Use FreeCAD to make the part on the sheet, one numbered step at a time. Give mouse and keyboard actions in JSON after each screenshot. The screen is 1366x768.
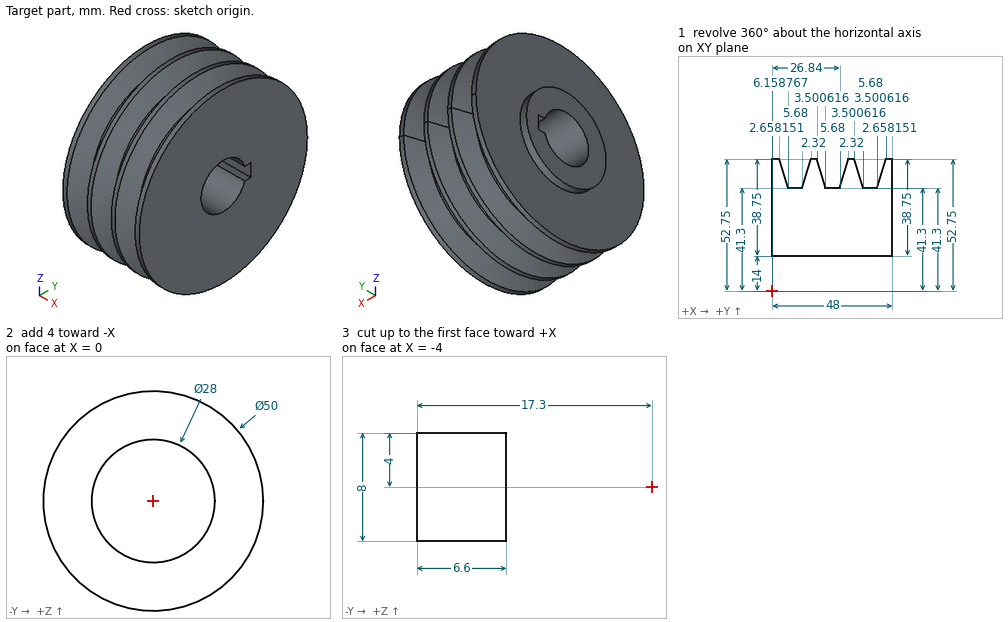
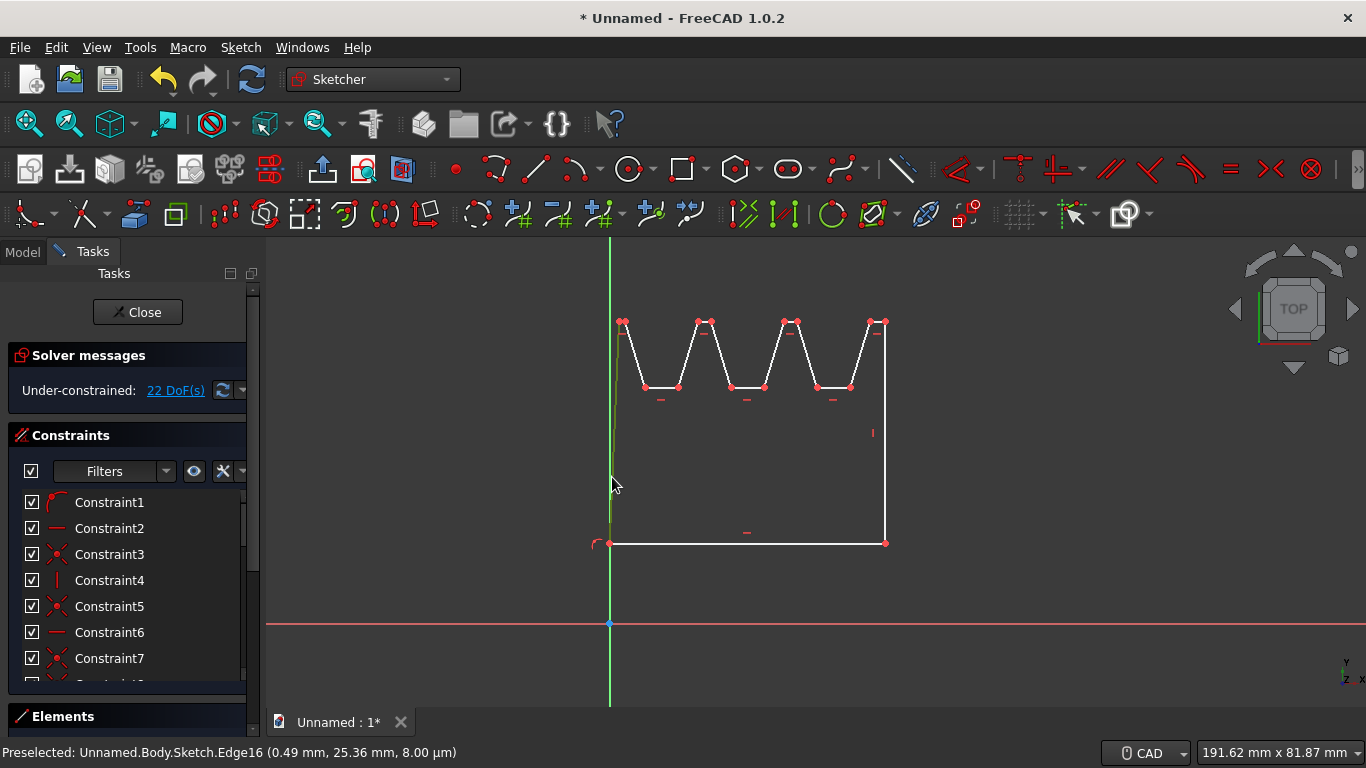
{"action": "key", "text": "v"}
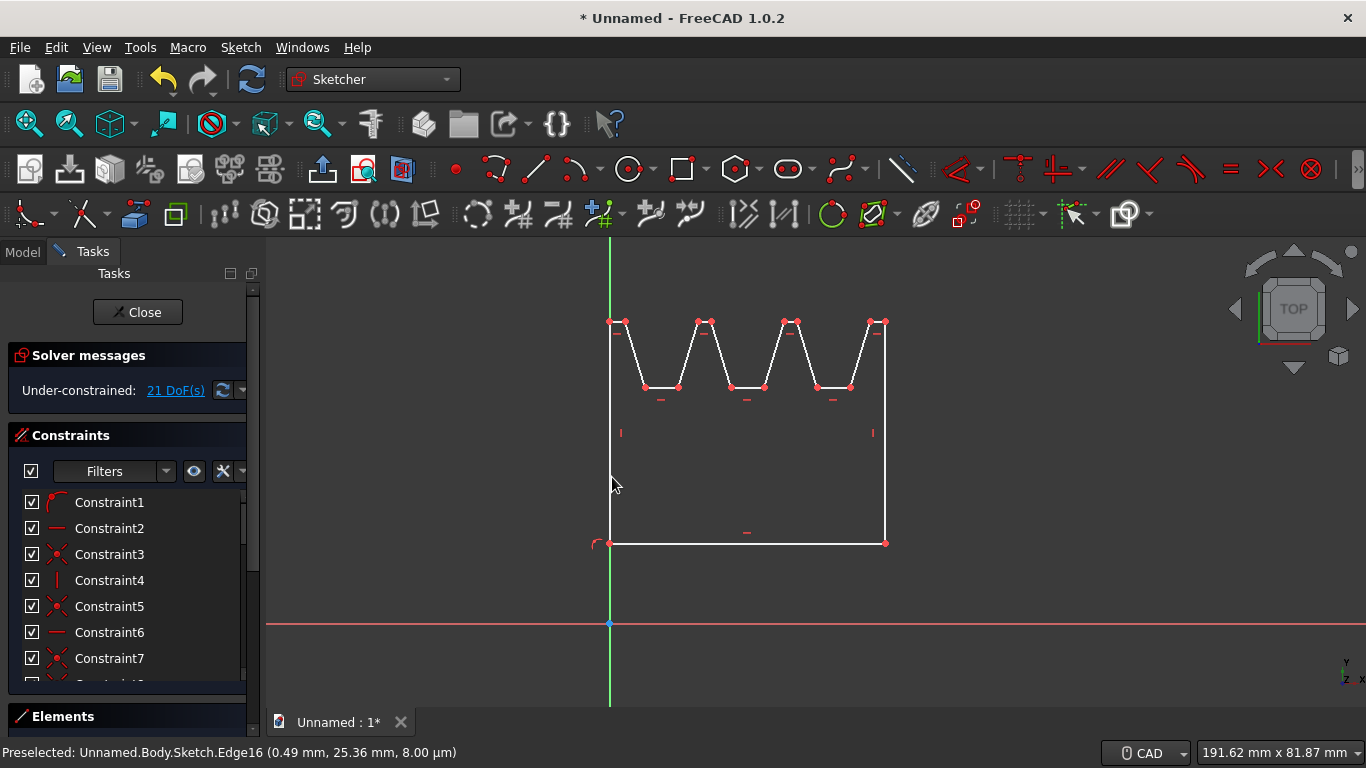
{"action": "left_click", "coordinate": [956, 170]}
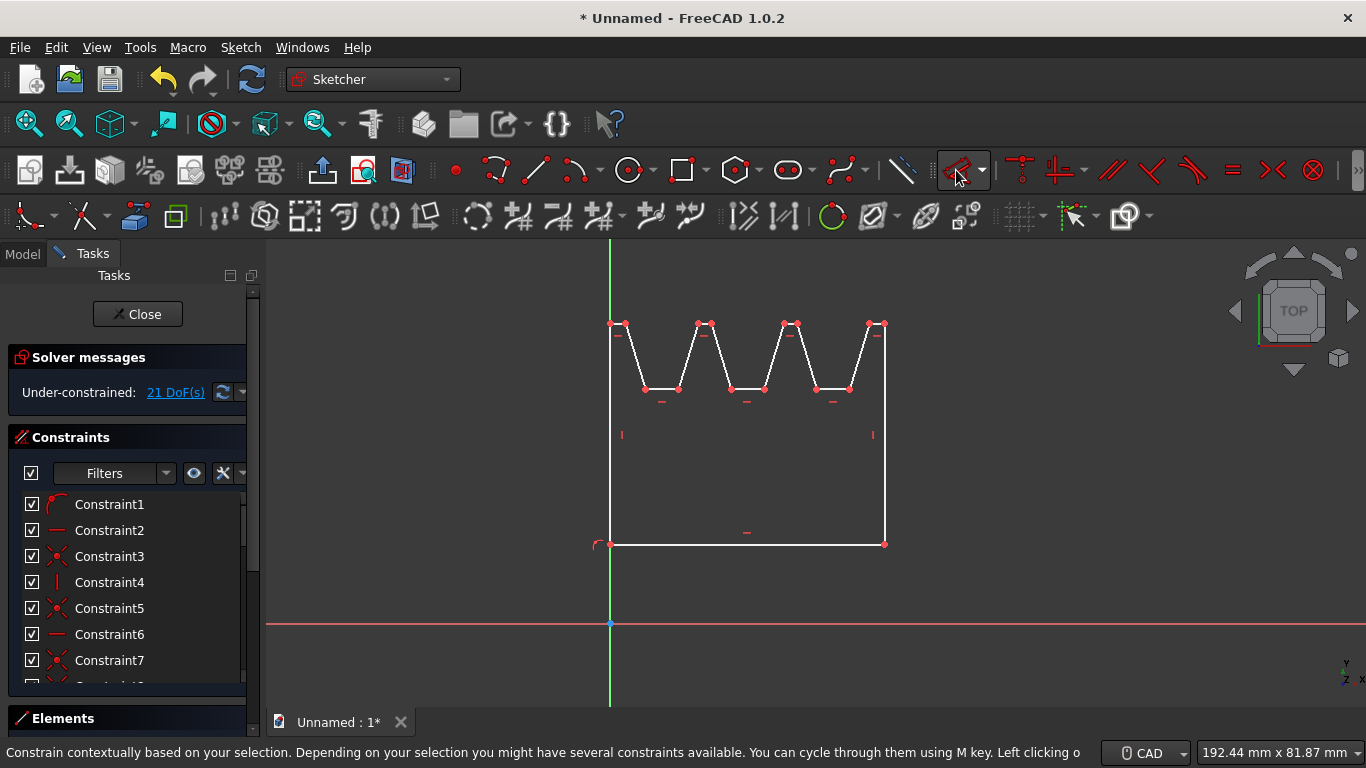
{"action": "left_click", "coordinate": [693, 545]}
{"action": "left_click", "coordinate": [748, 579]}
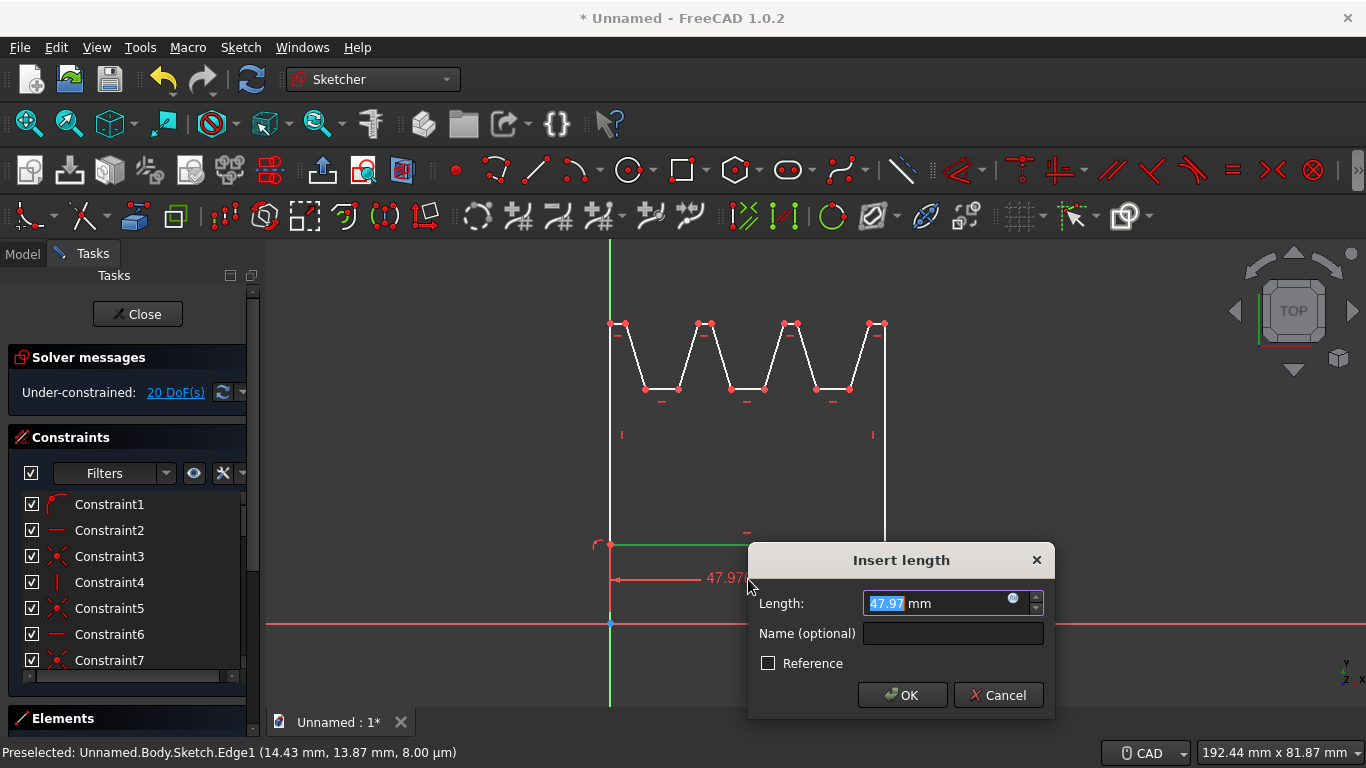
{"action": "type", "text": "48"}
{"action": "key", "text": "Return"}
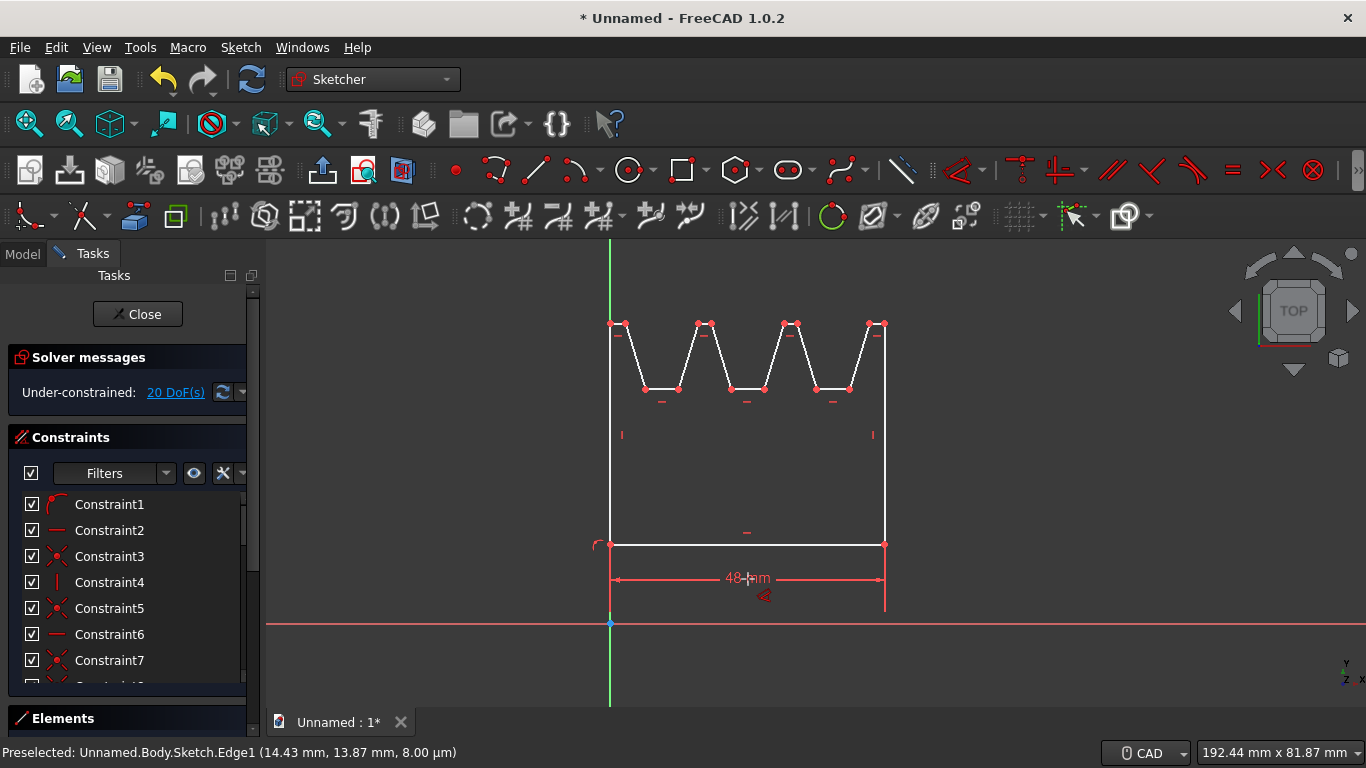
{"action": "left_click", "coordinate": [610, 545]}
{"action": "left_click", "coordinate": [576, 584]}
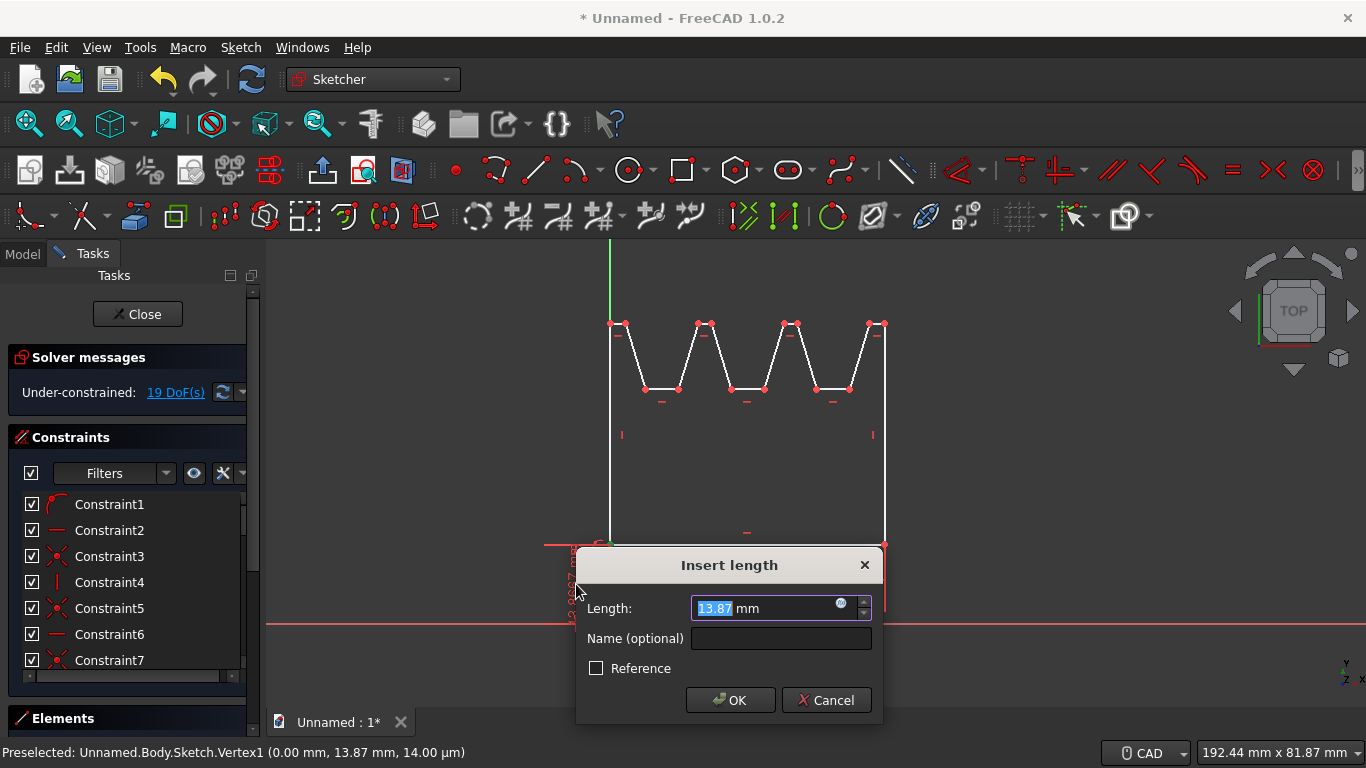
{"action": "type", "text": "14"}
{"action": "key", "text": "Return"}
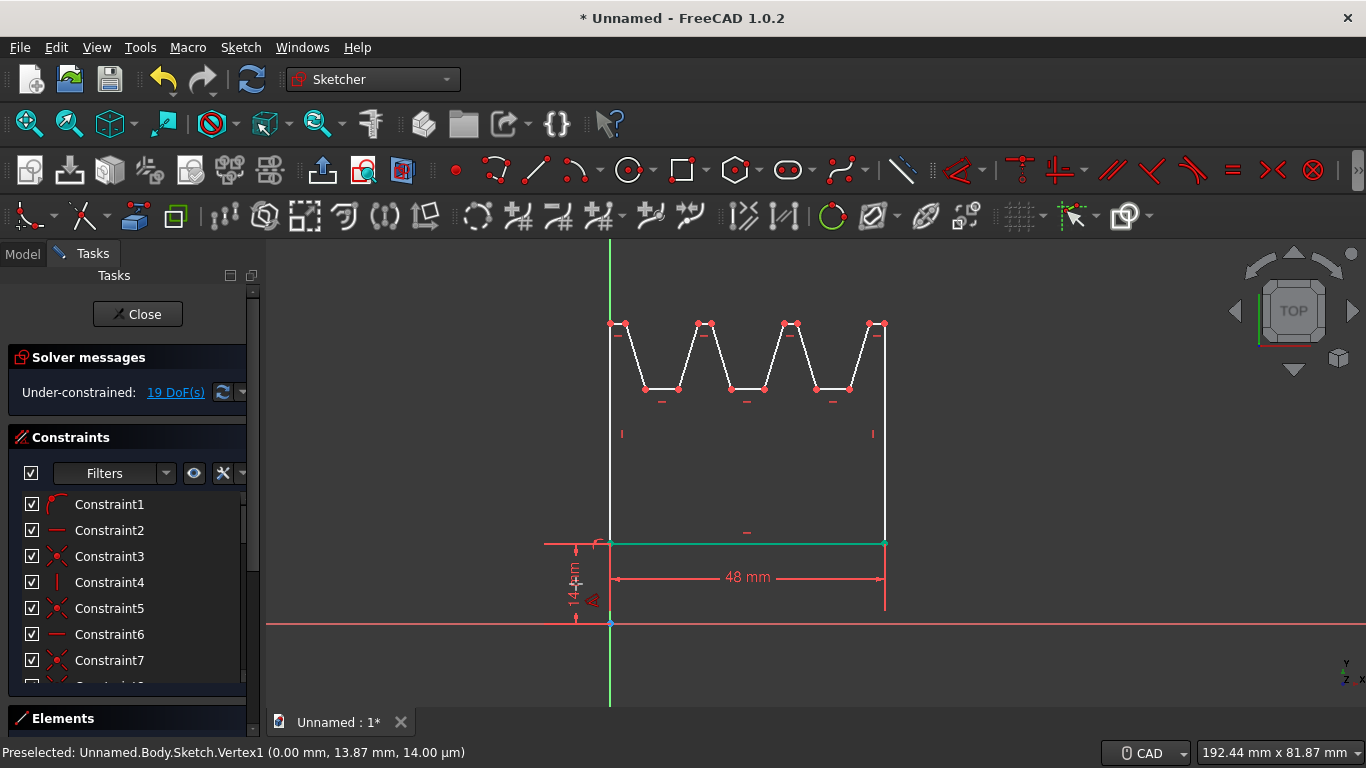
{"action": "scroll", "coordinate": [840, 389], "scroll_direction": "up", "scroll_amount": 2}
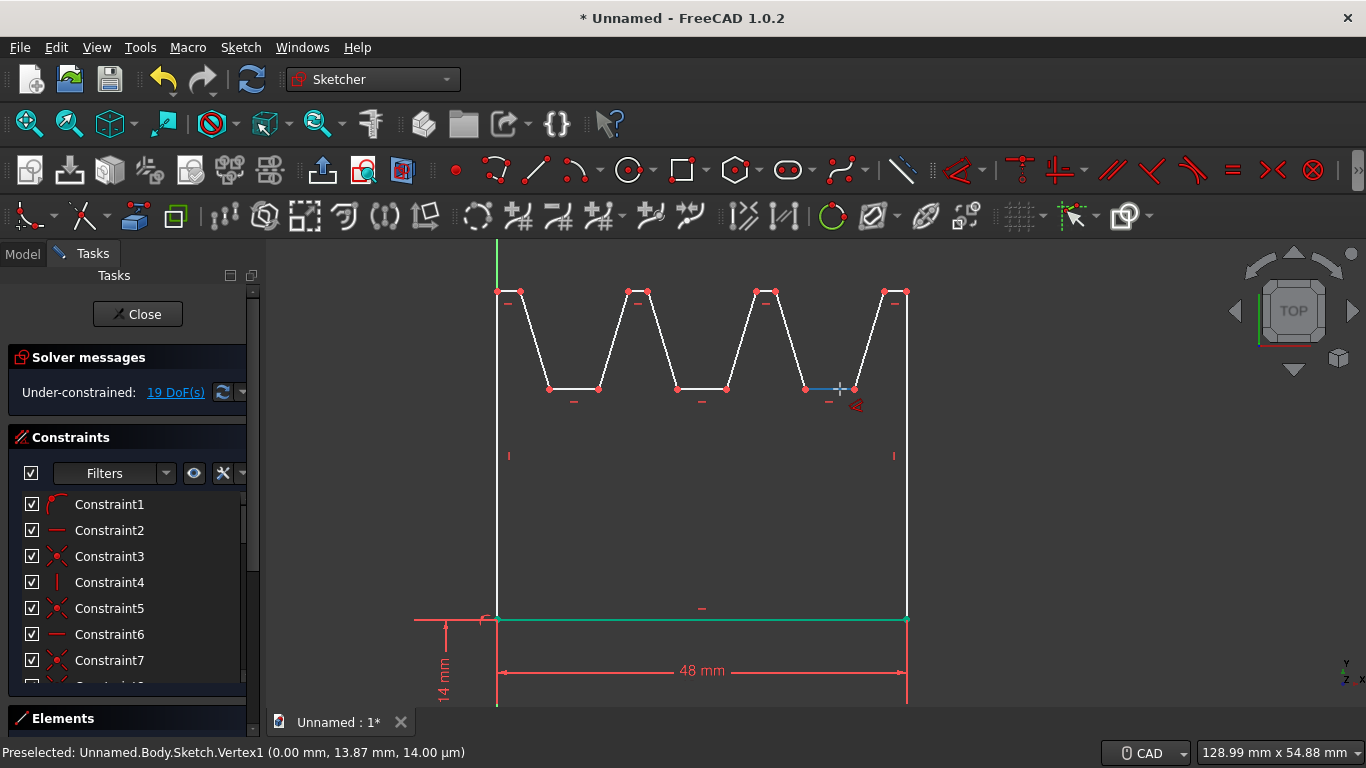
{"action": "left_click", "coordinate": [840, 389]}
{"action": "left_click", "coordinate": [830, 355]}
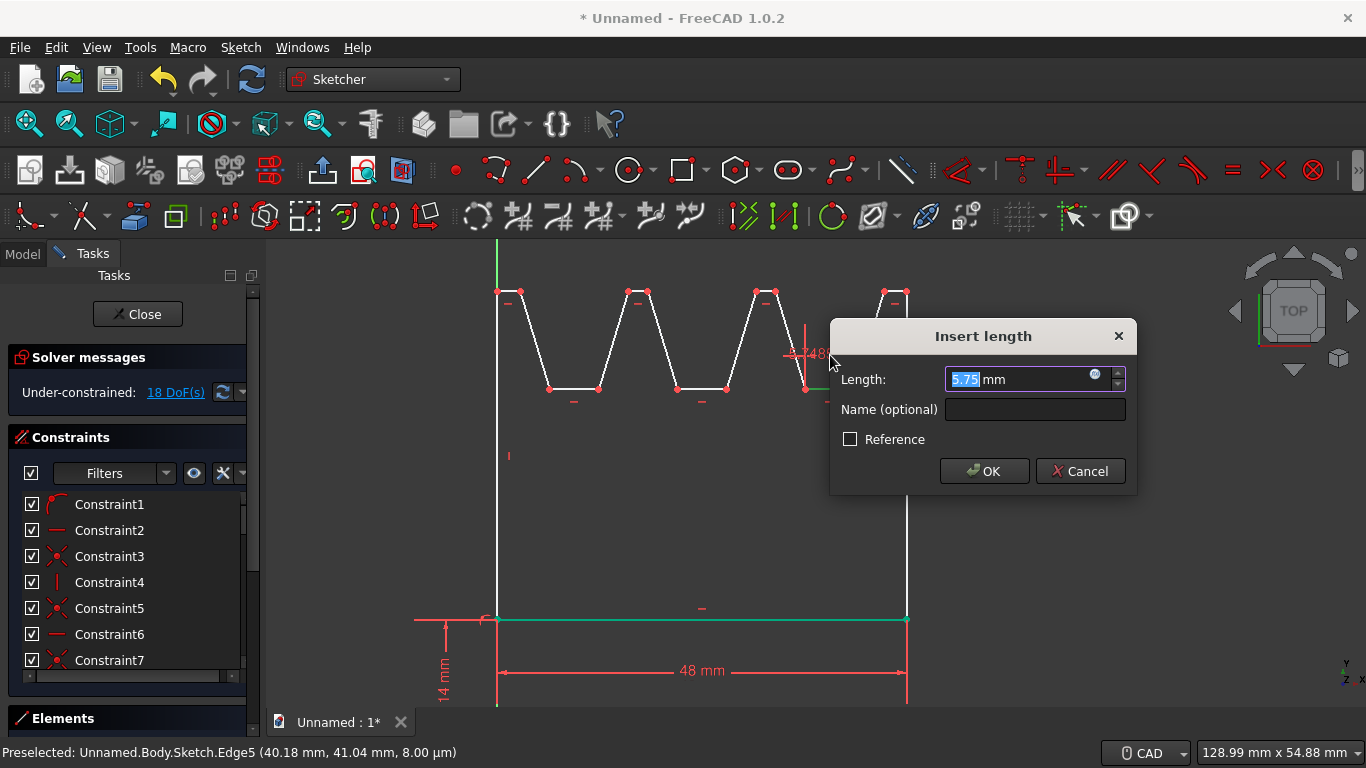
{"action": "type", "text": "5.68"}
{"action": "key", "text": "Return"}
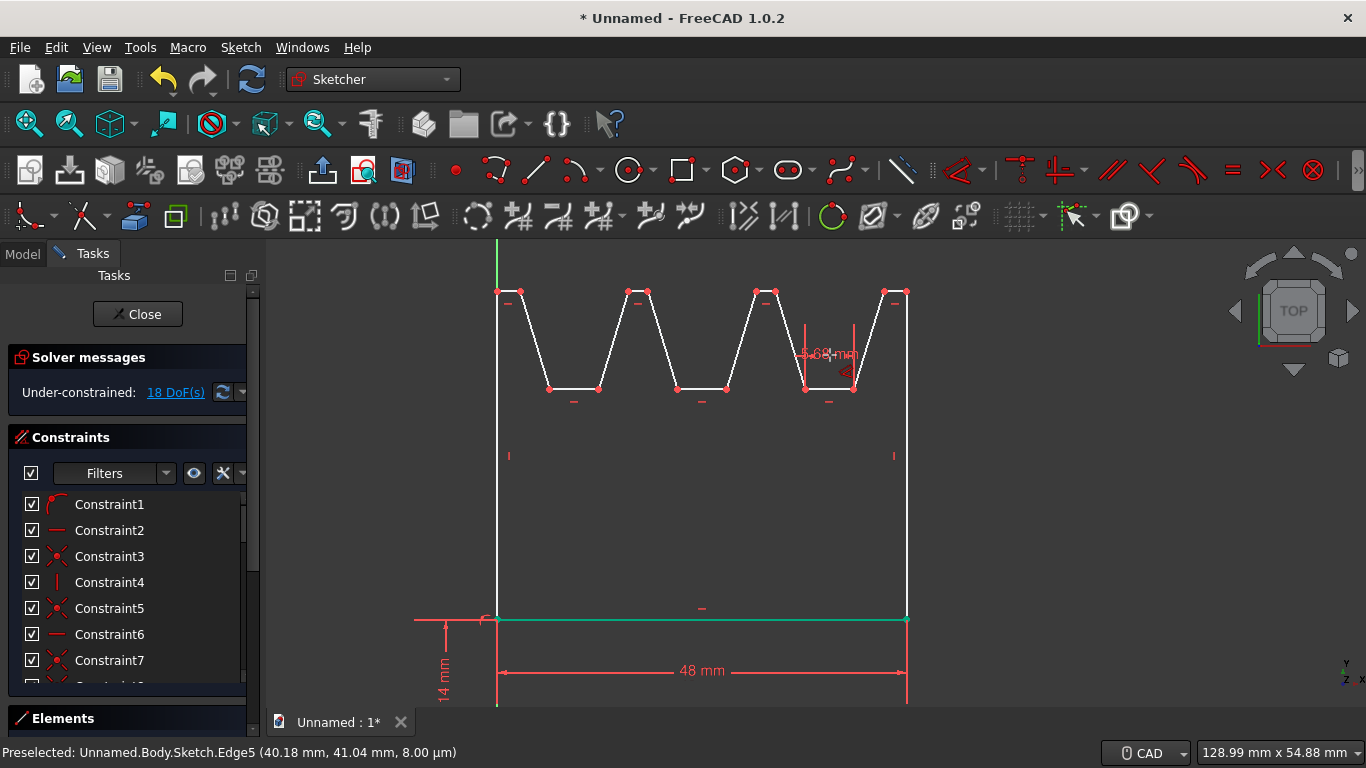
{"action": "scroll", "coordinate": [766, 291], "scroll_direction": "up", "scroll_amount": 4}